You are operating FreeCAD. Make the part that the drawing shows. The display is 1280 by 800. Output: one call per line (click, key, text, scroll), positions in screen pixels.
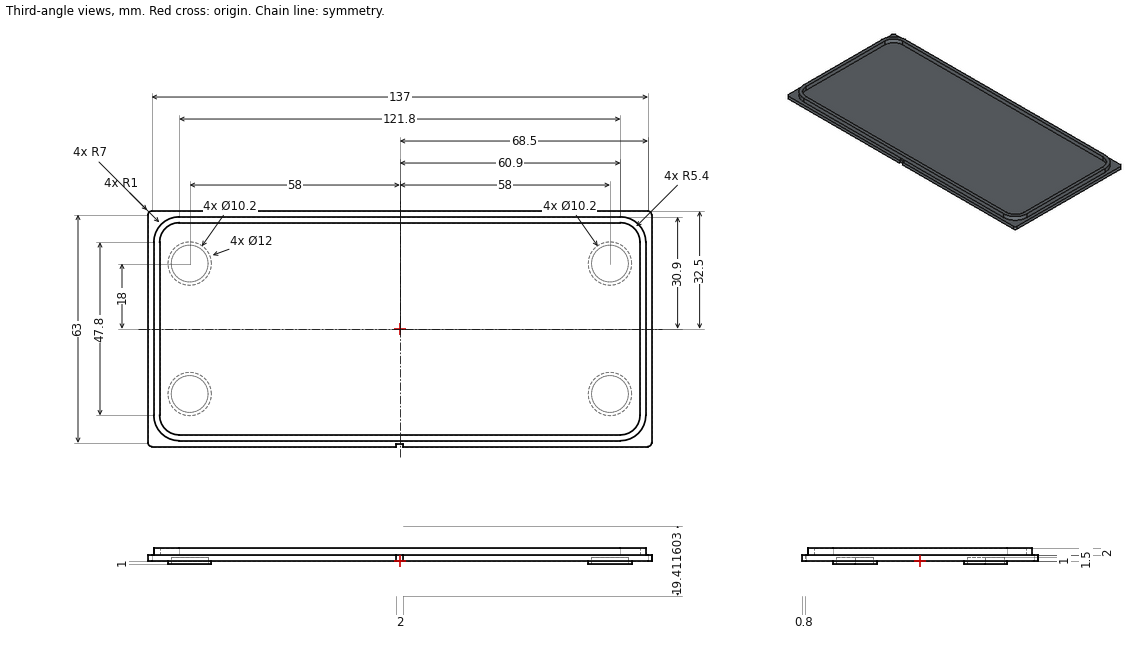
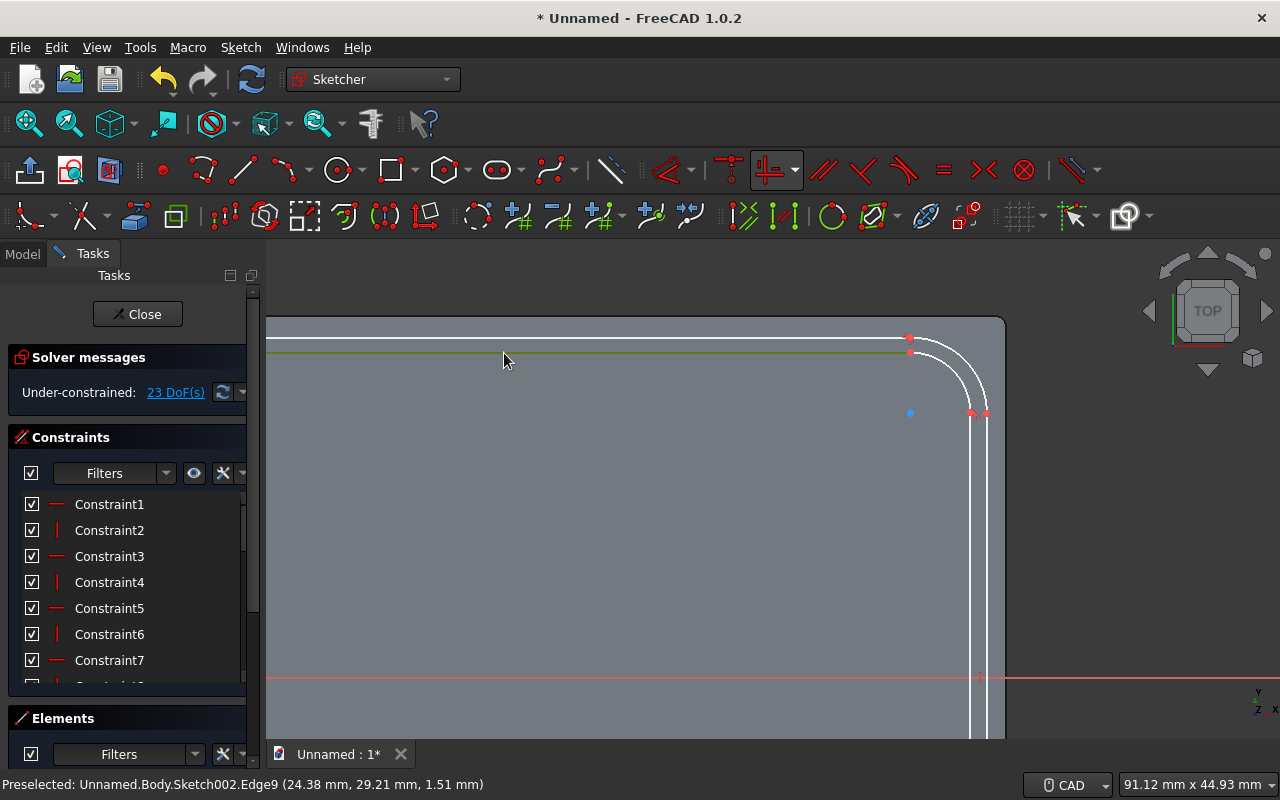
scroll(979, 379, down, 5)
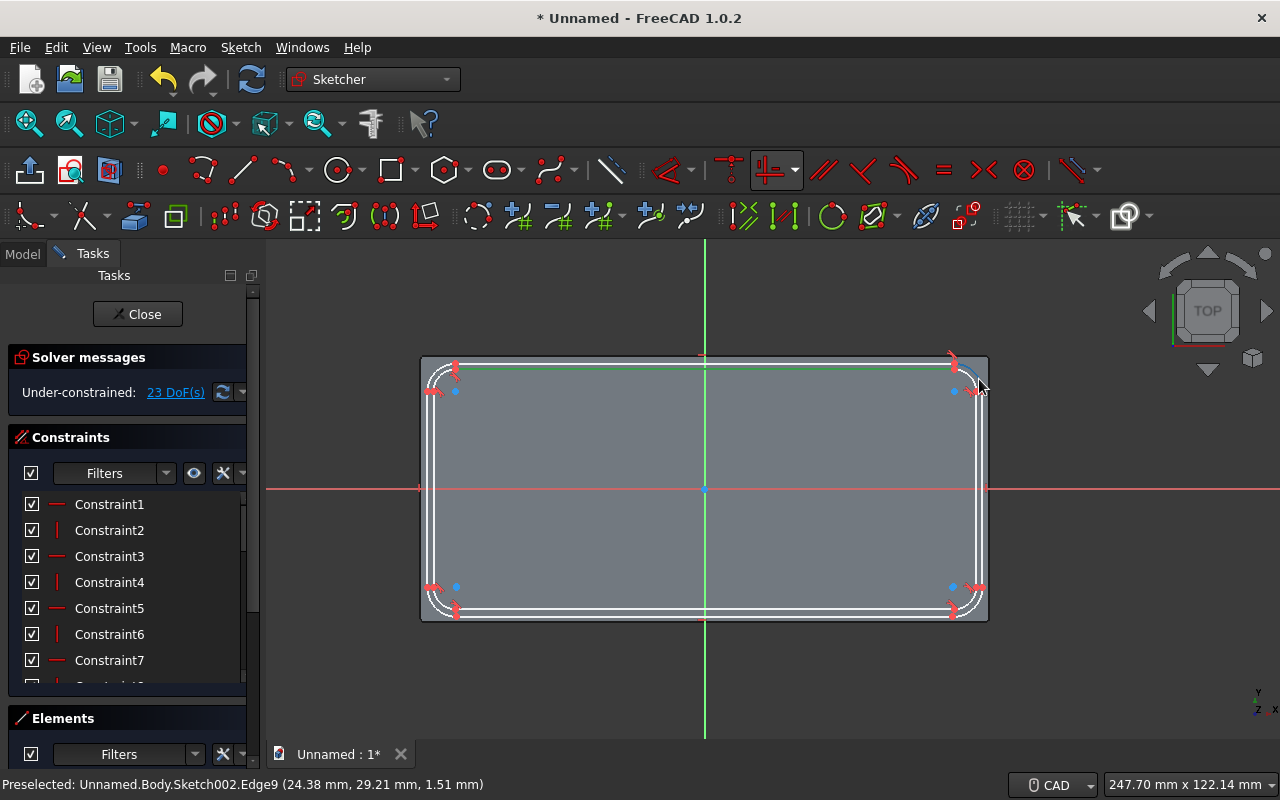
scroll(446, 372, up, 5)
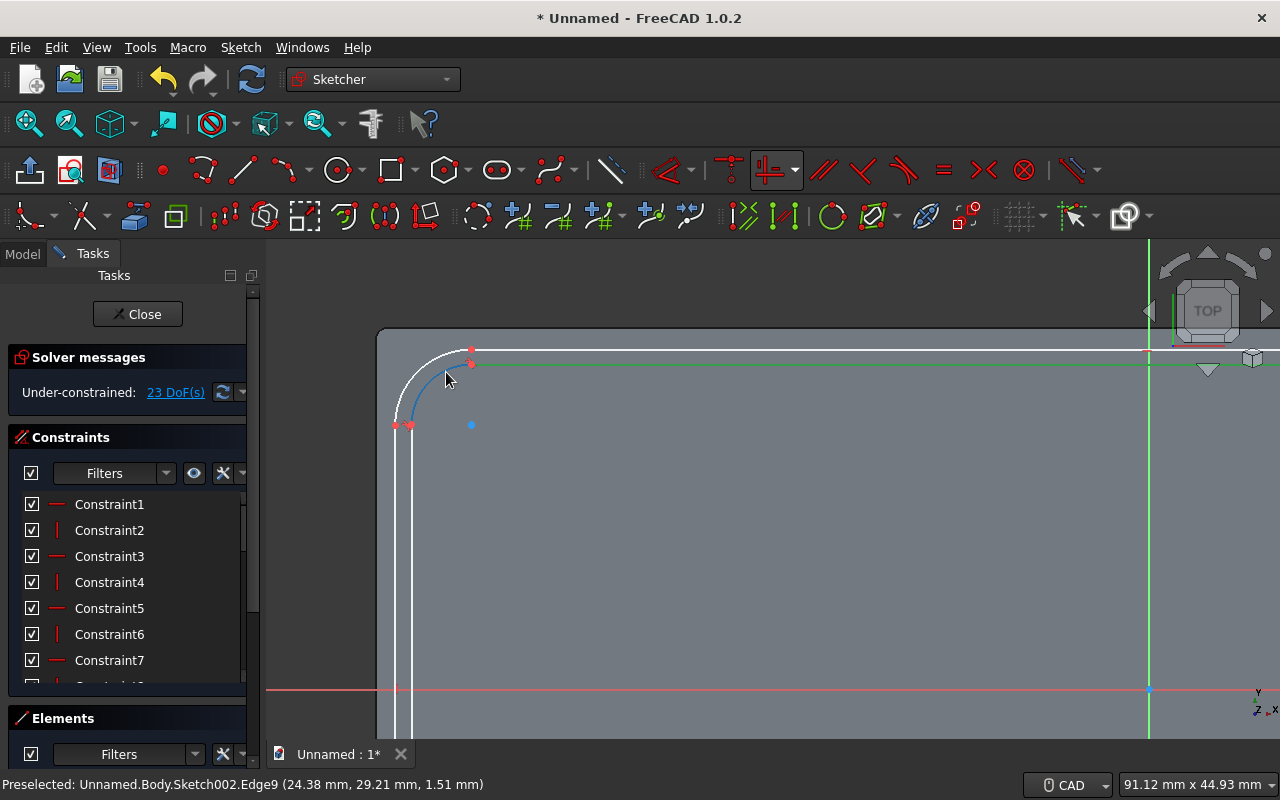
click(445, 371)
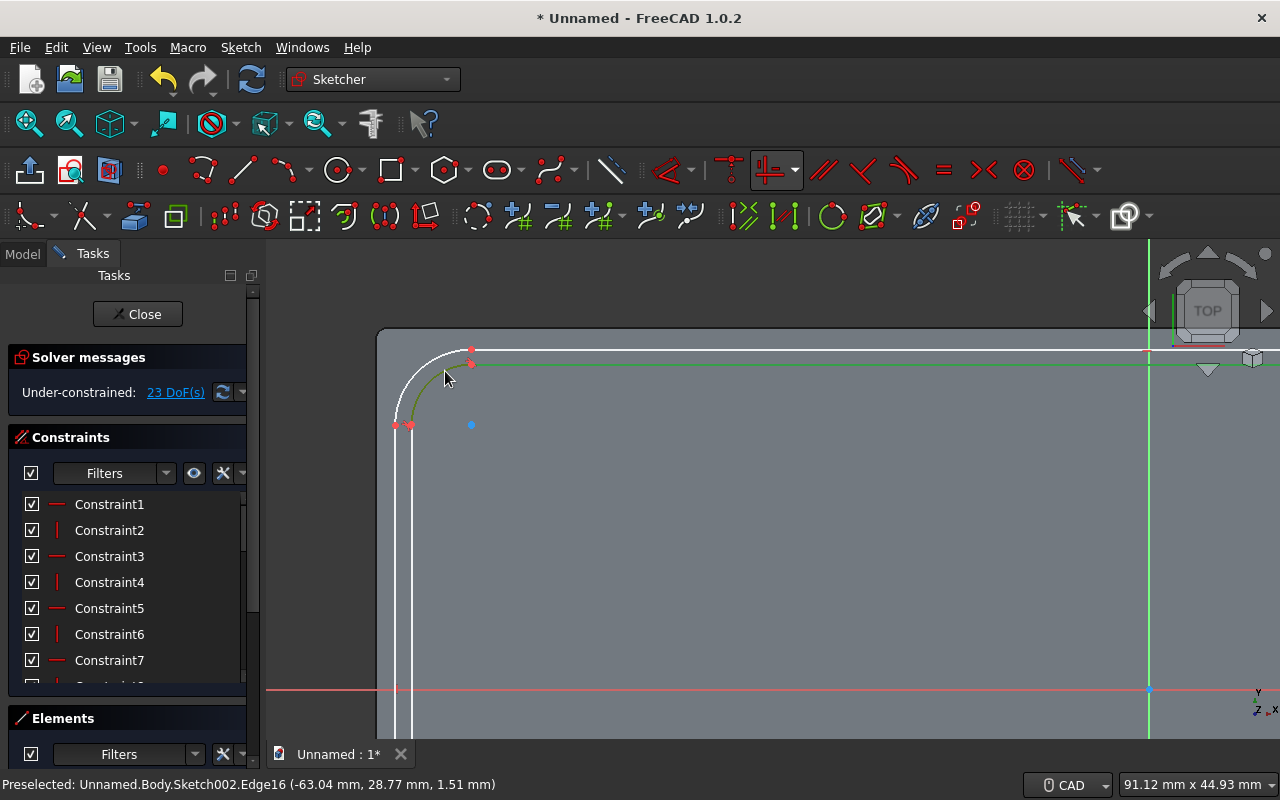
click(904, 170)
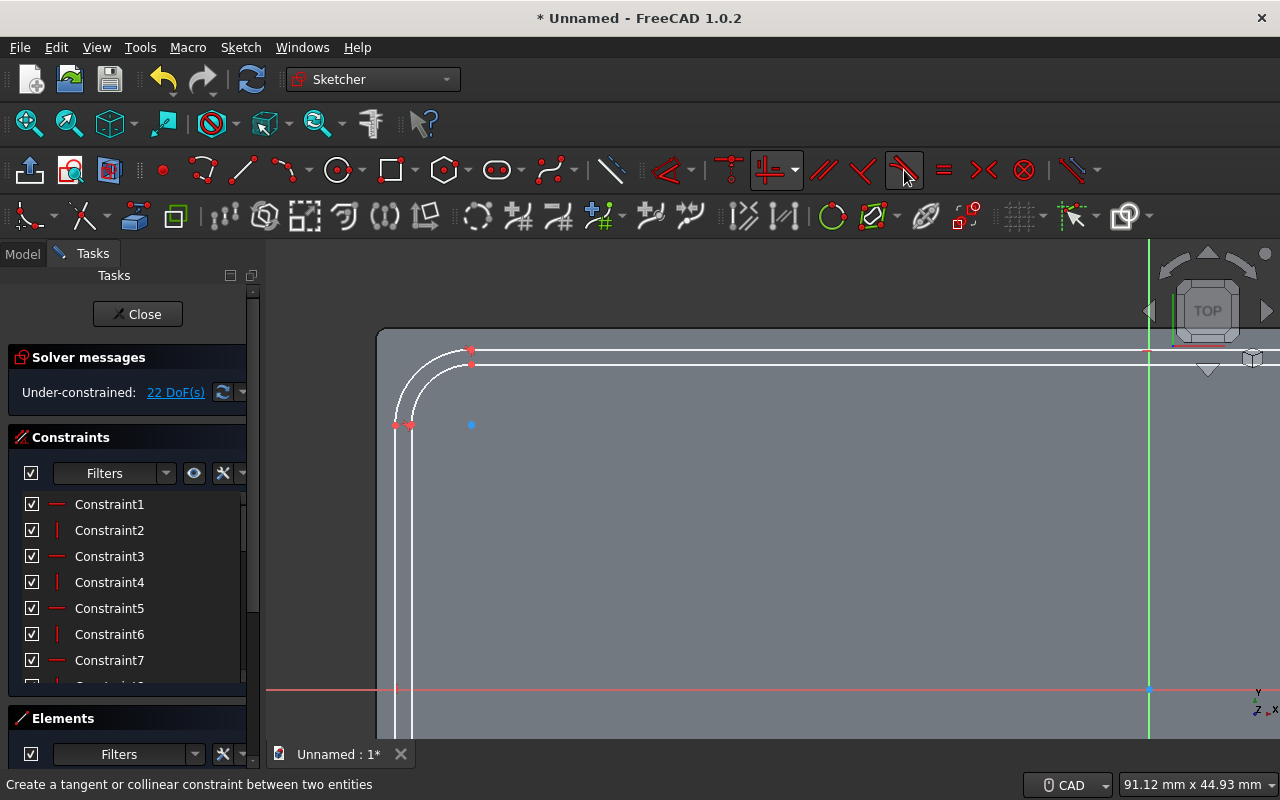
scroll(446, 372, down, 5)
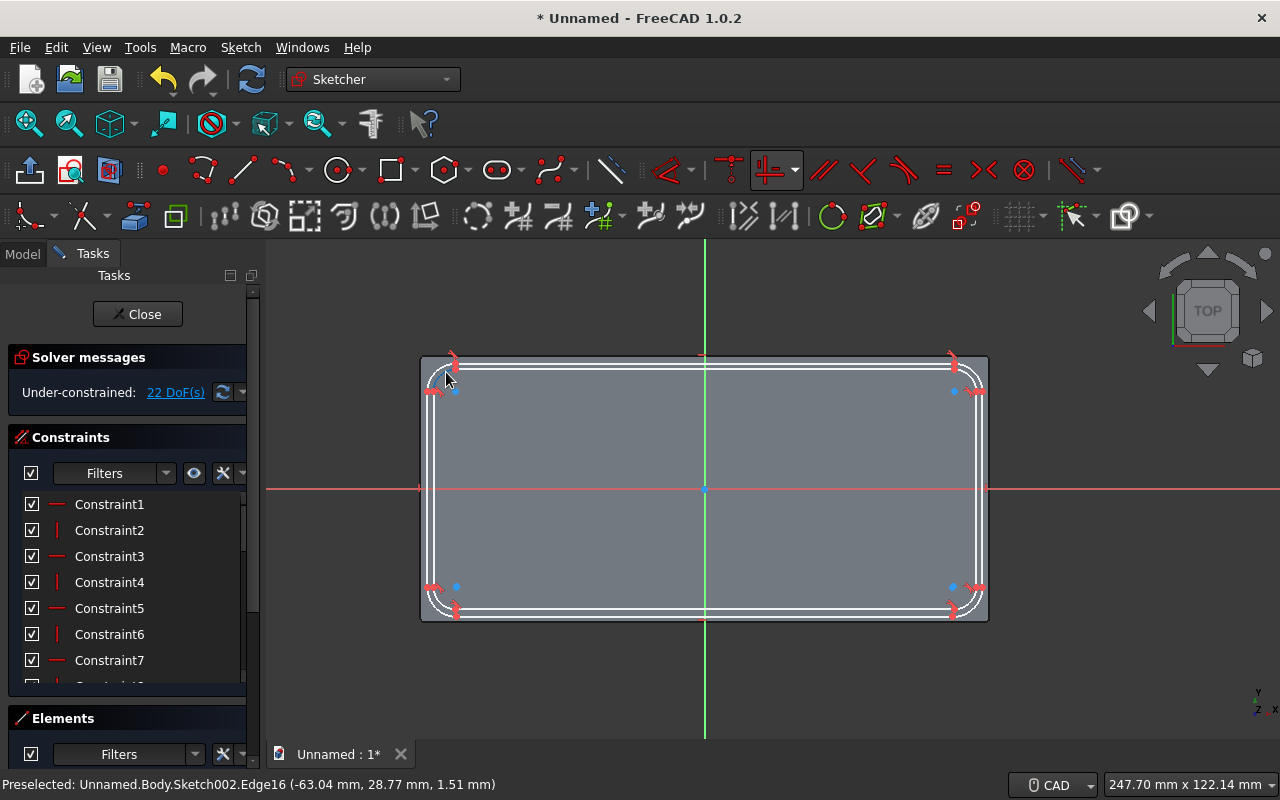
scroll(976, 450, up, 5)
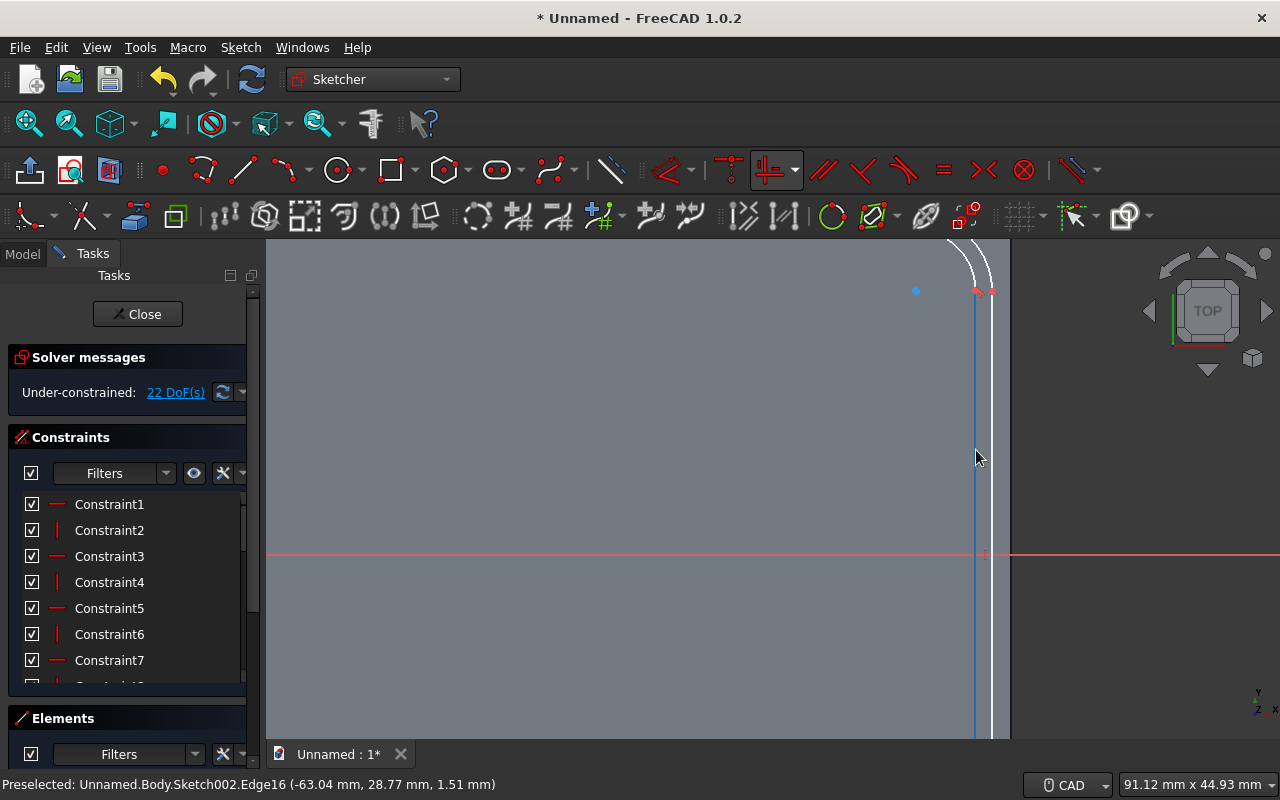
click(975, 450)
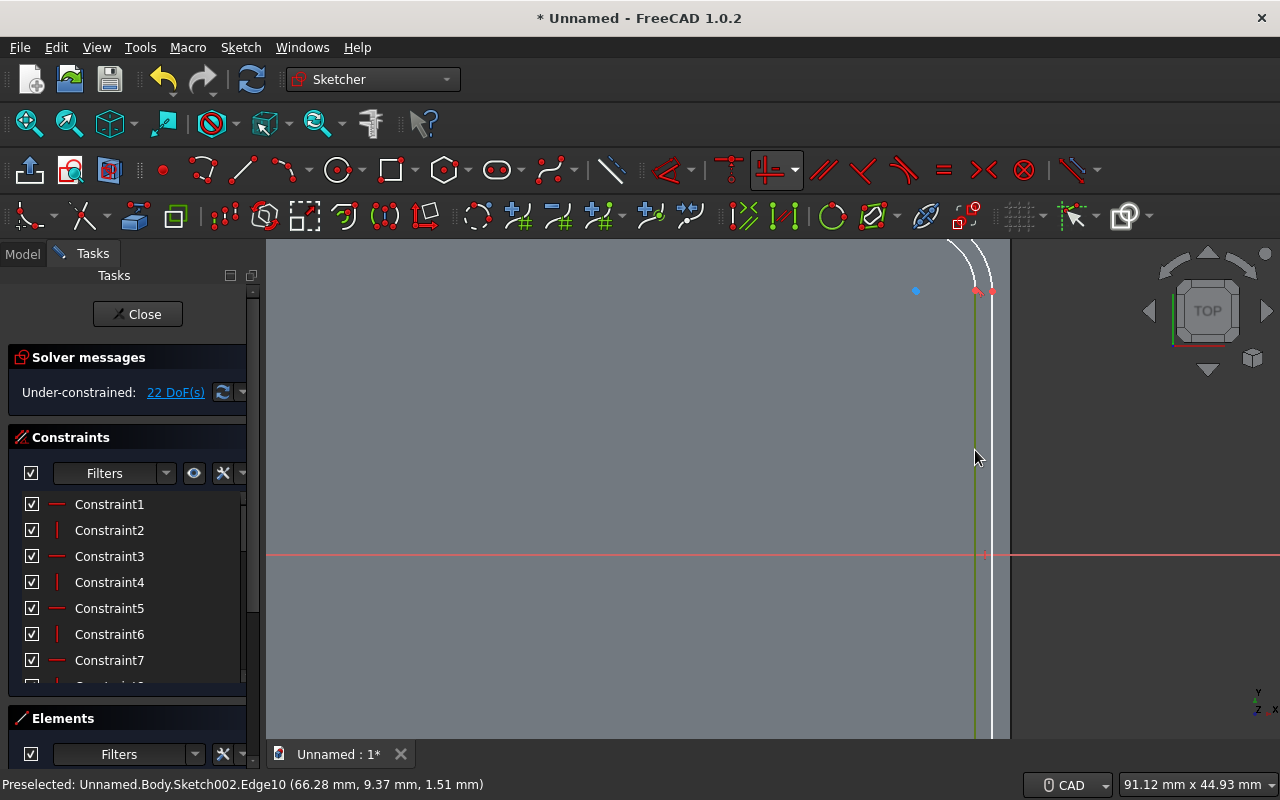
click(973, 272)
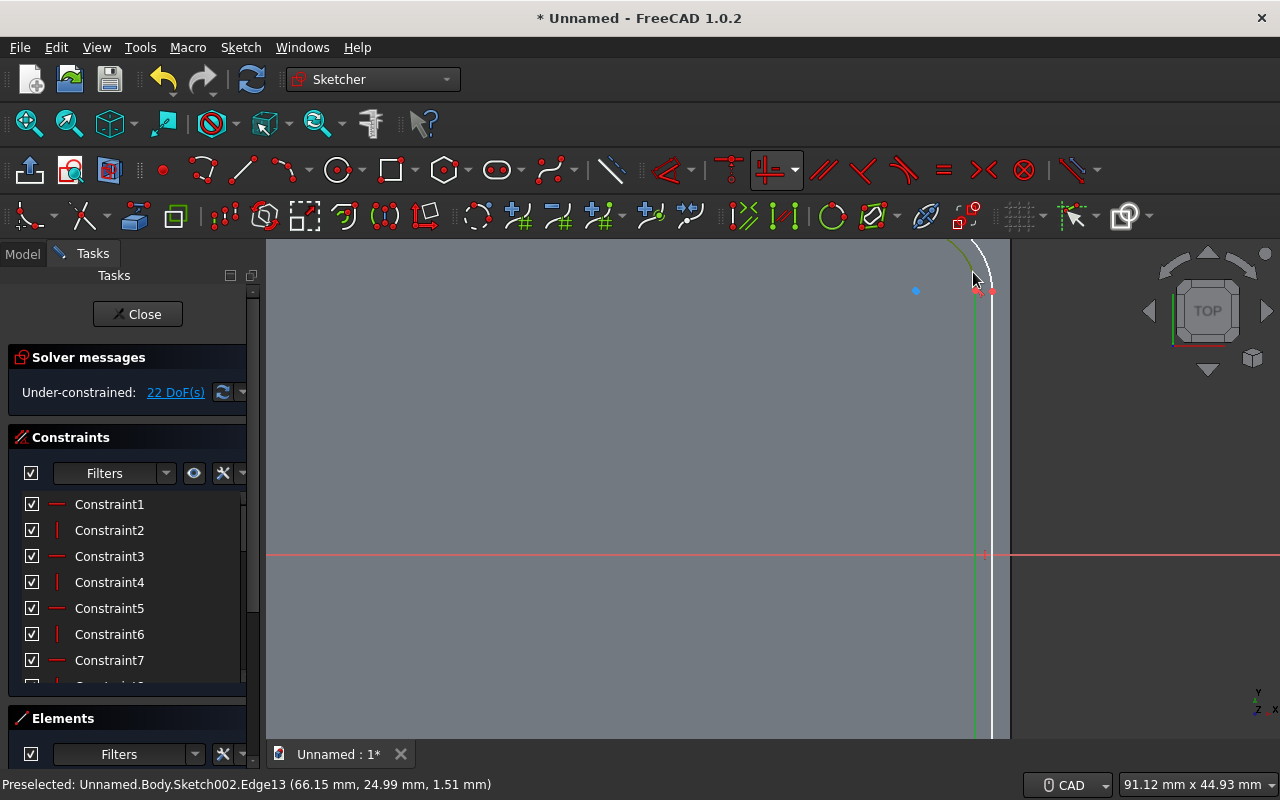
click(904, 170)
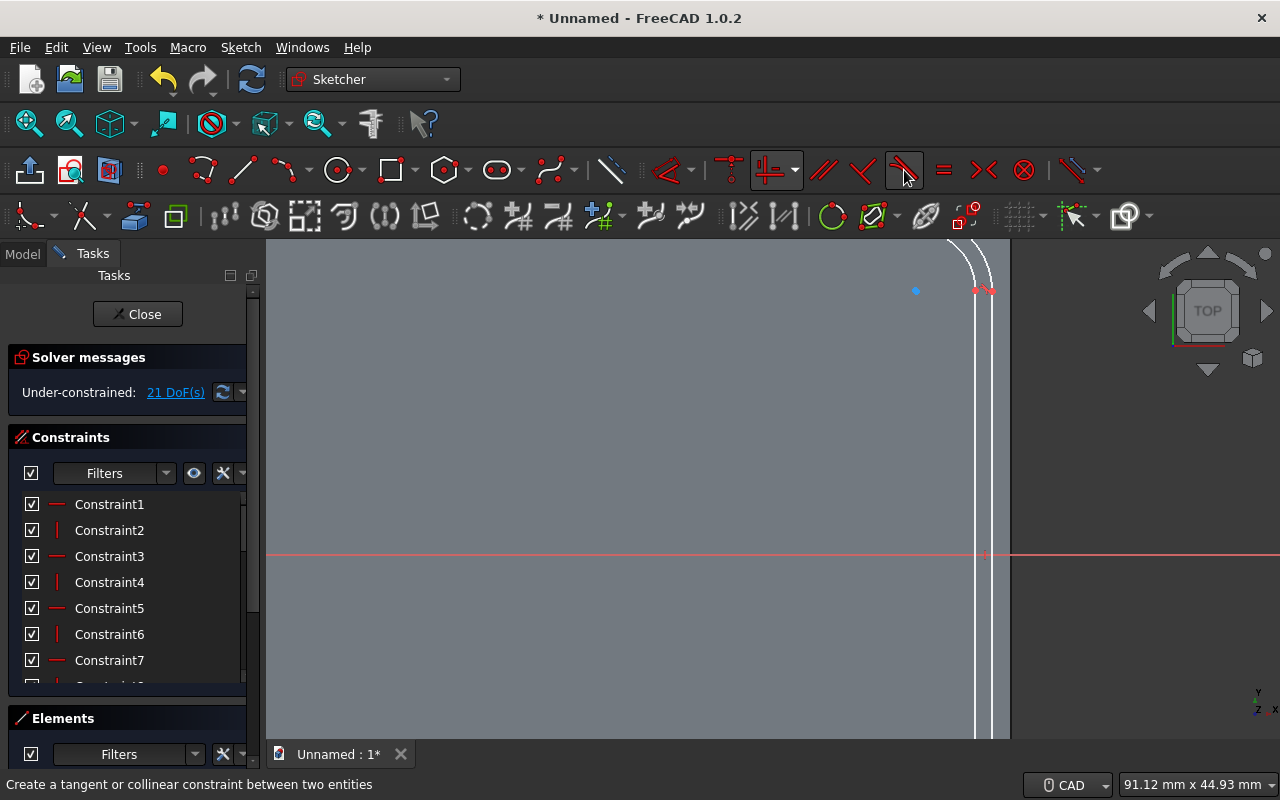
click(975, 450)